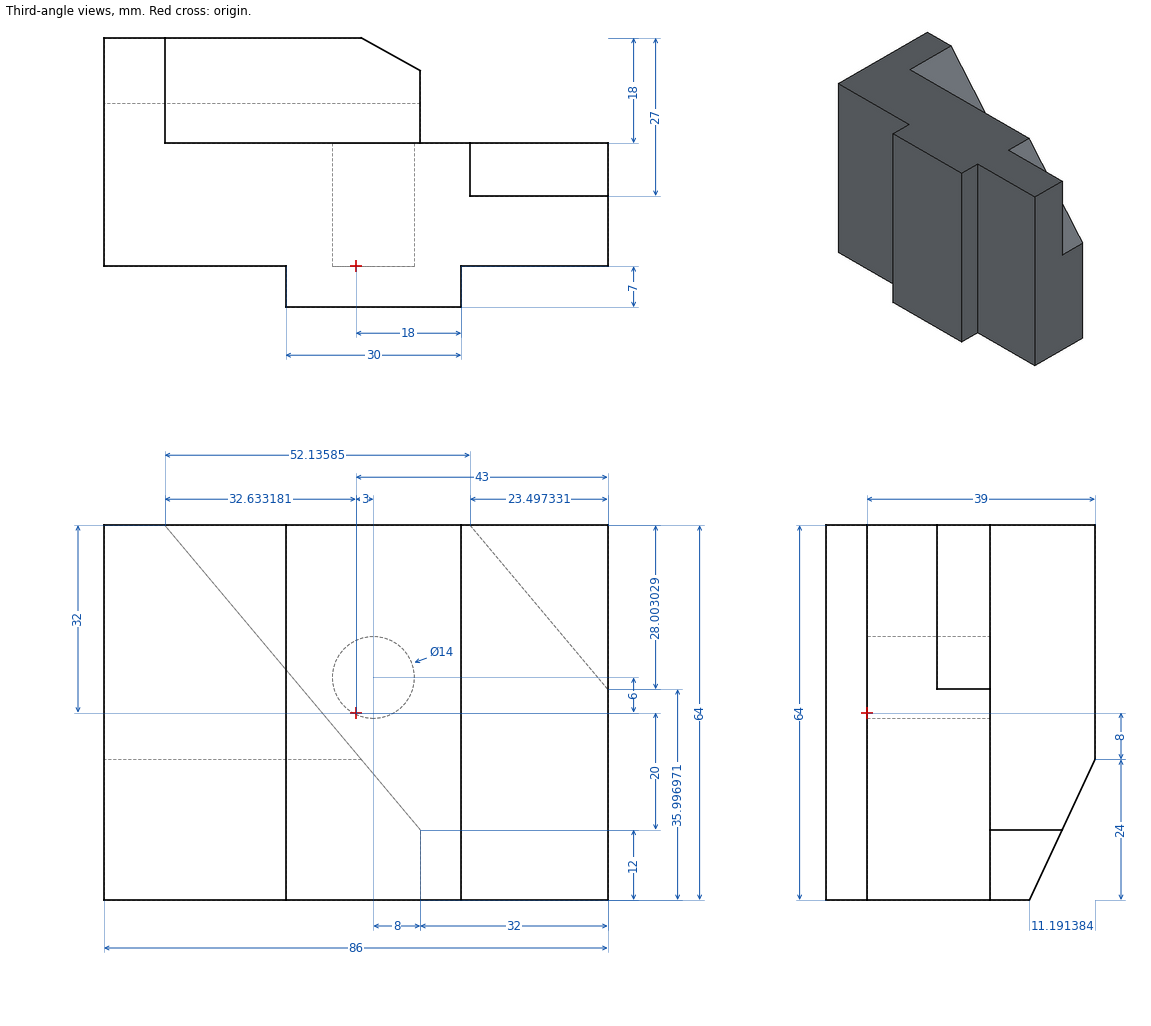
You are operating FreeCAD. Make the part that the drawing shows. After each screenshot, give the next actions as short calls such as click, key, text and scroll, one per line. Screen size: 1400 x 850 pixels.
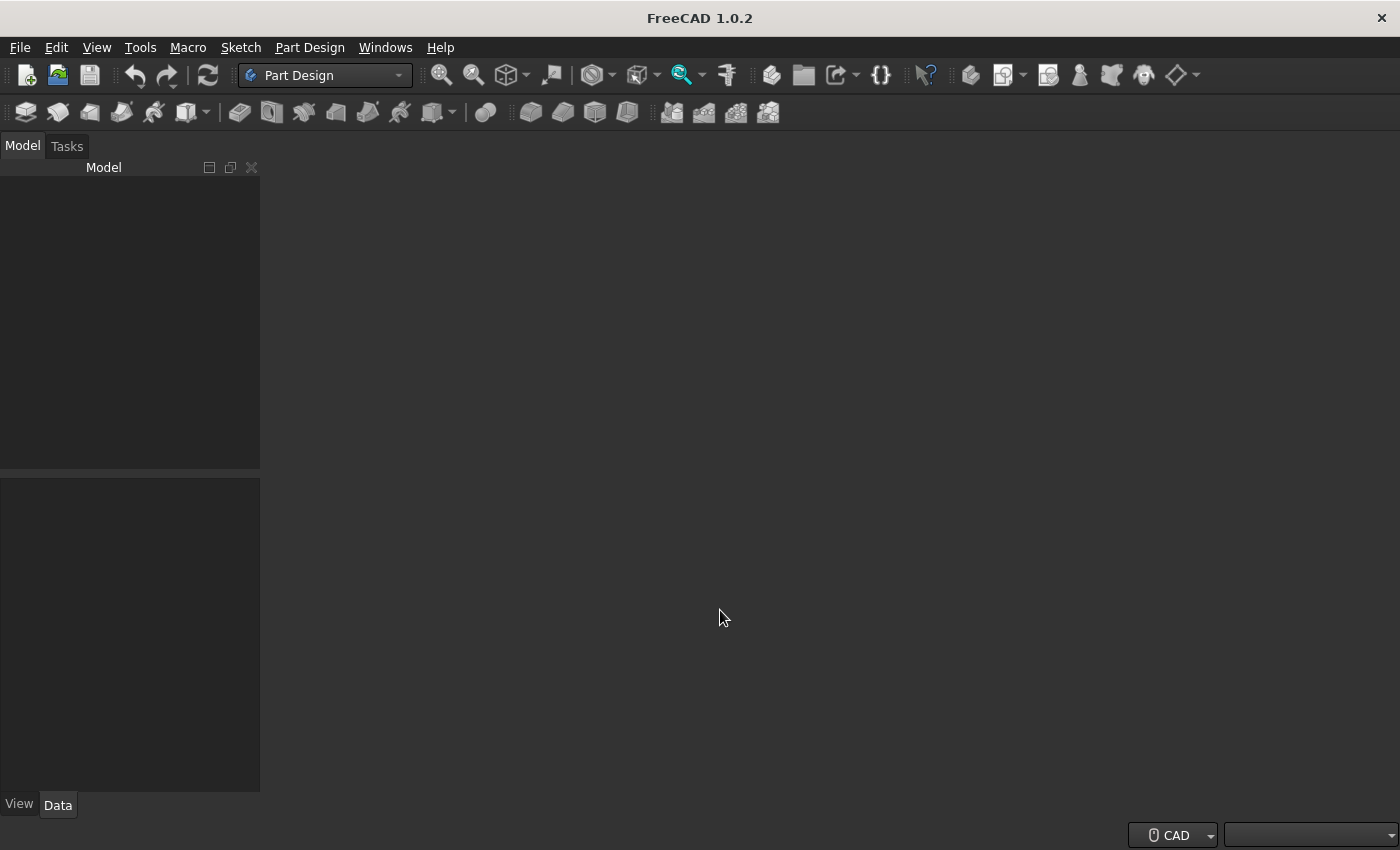
key(ctrl+n)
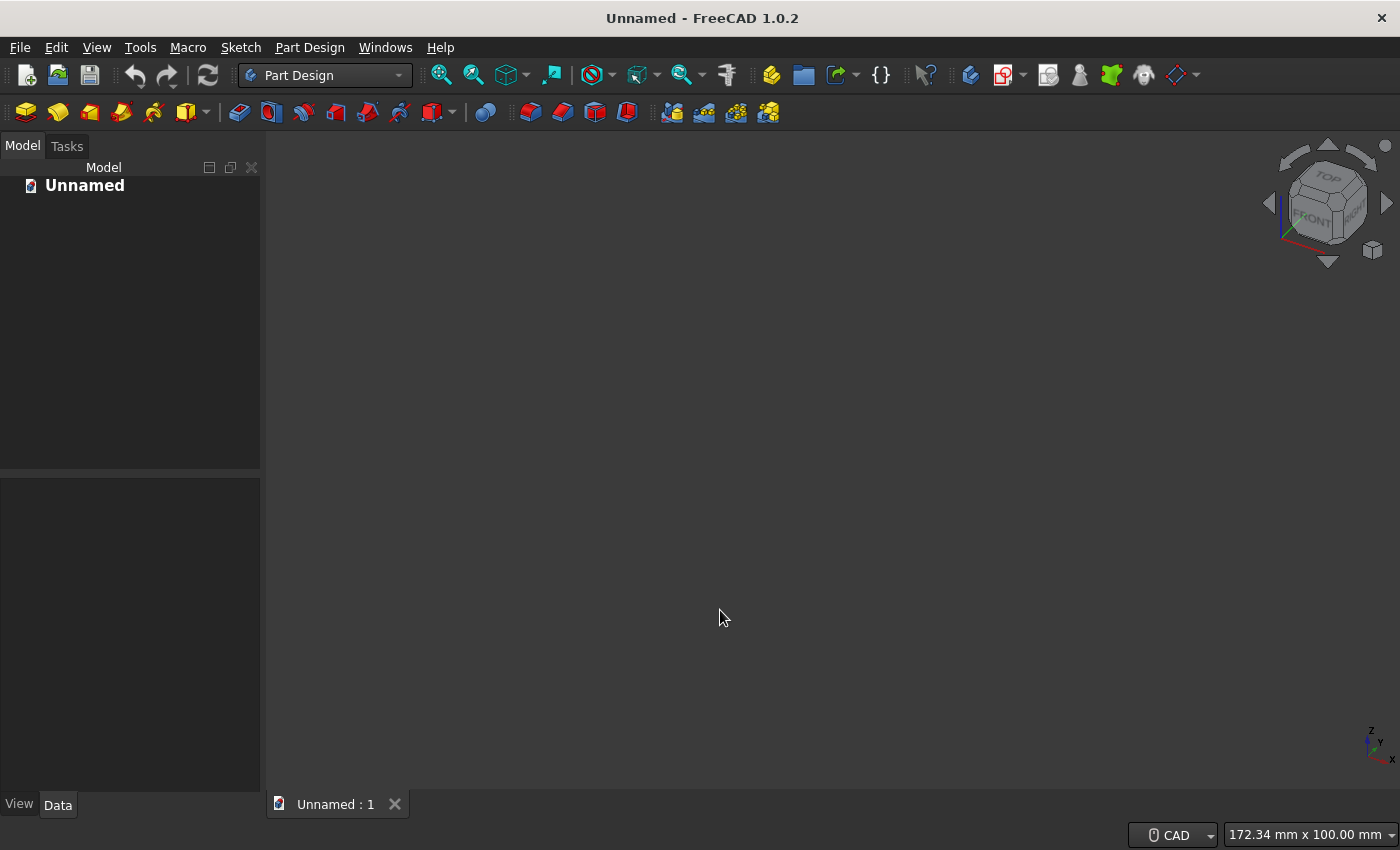
click(1004, 76)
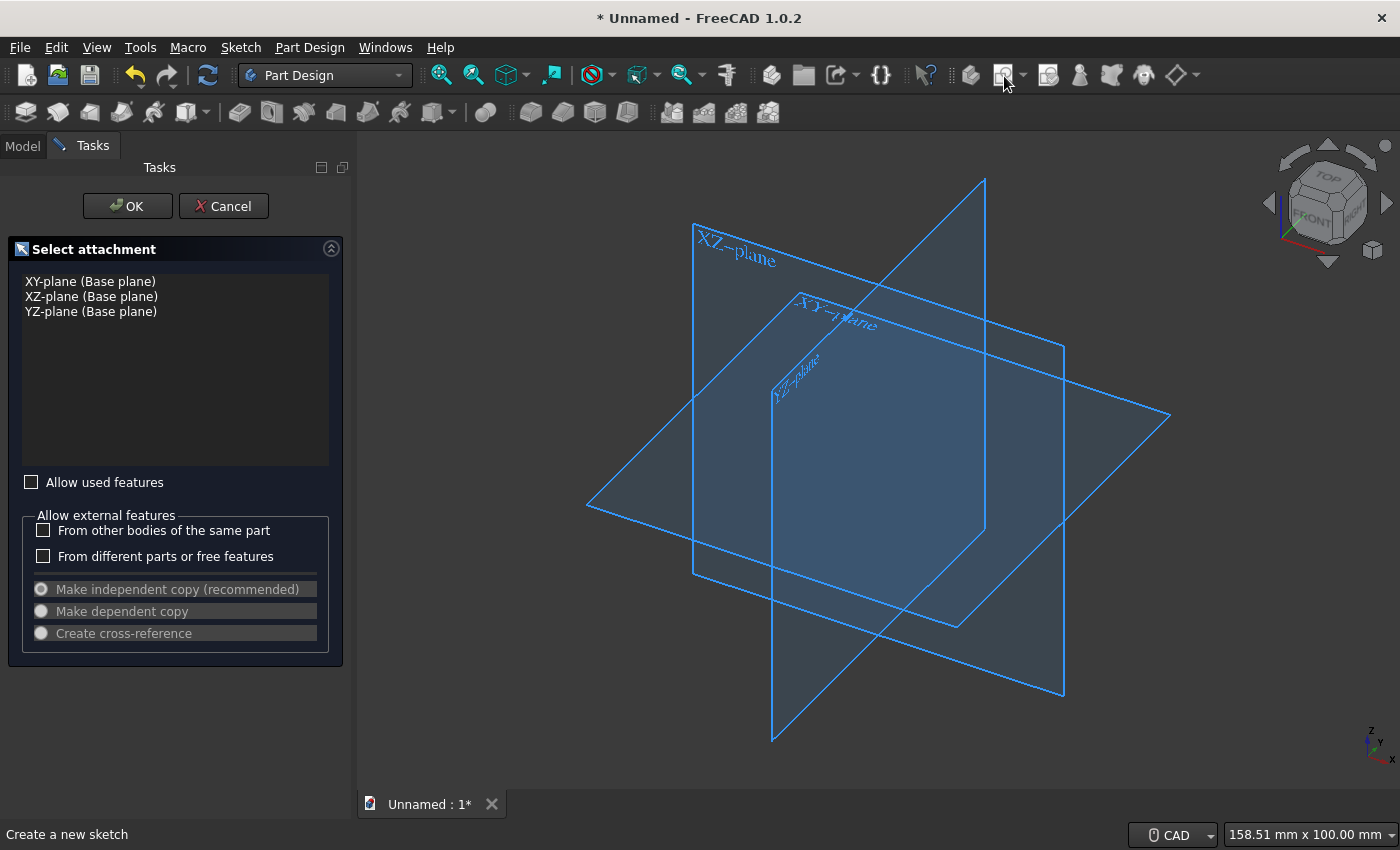
click(82, 296)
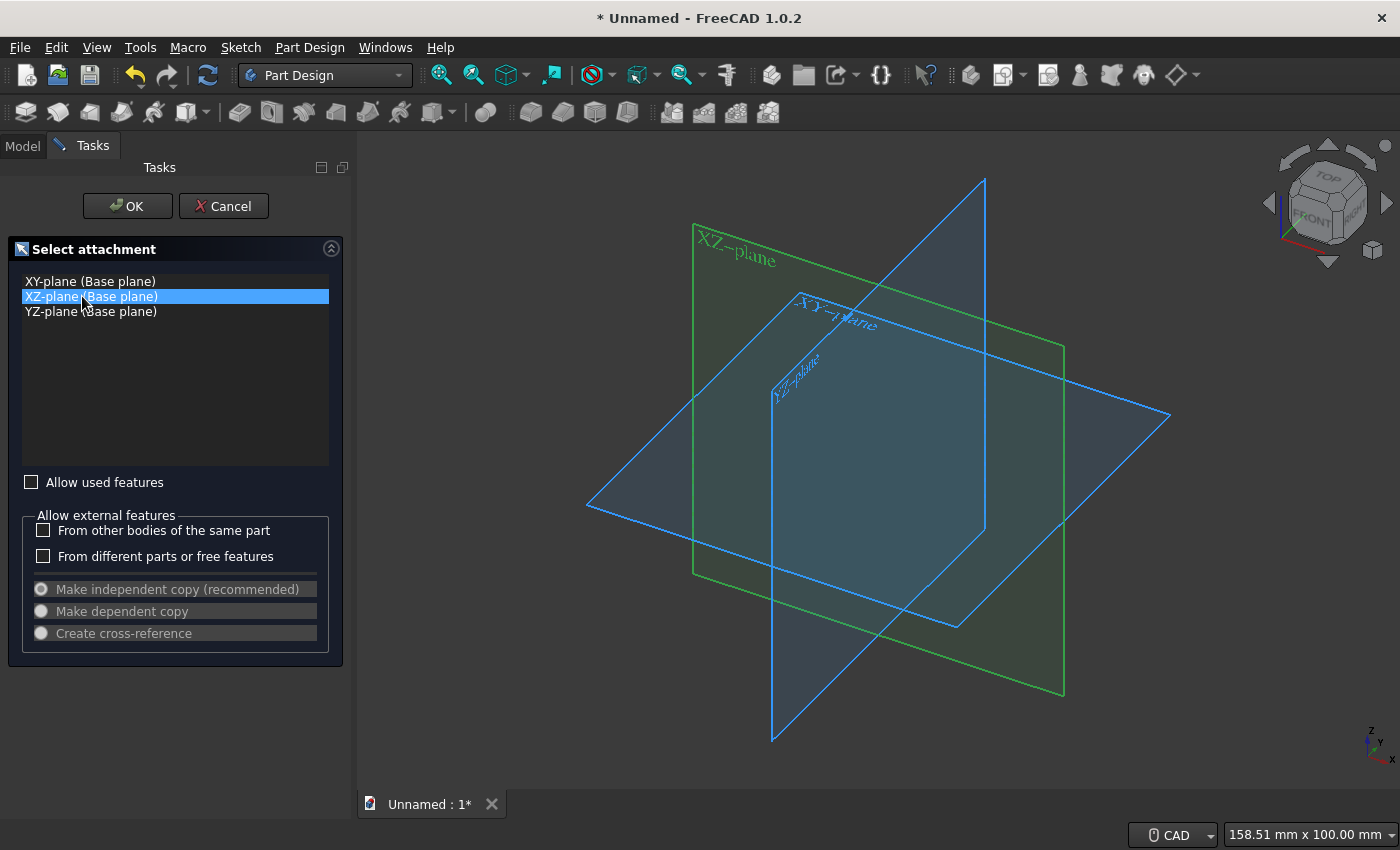
click(128, 206)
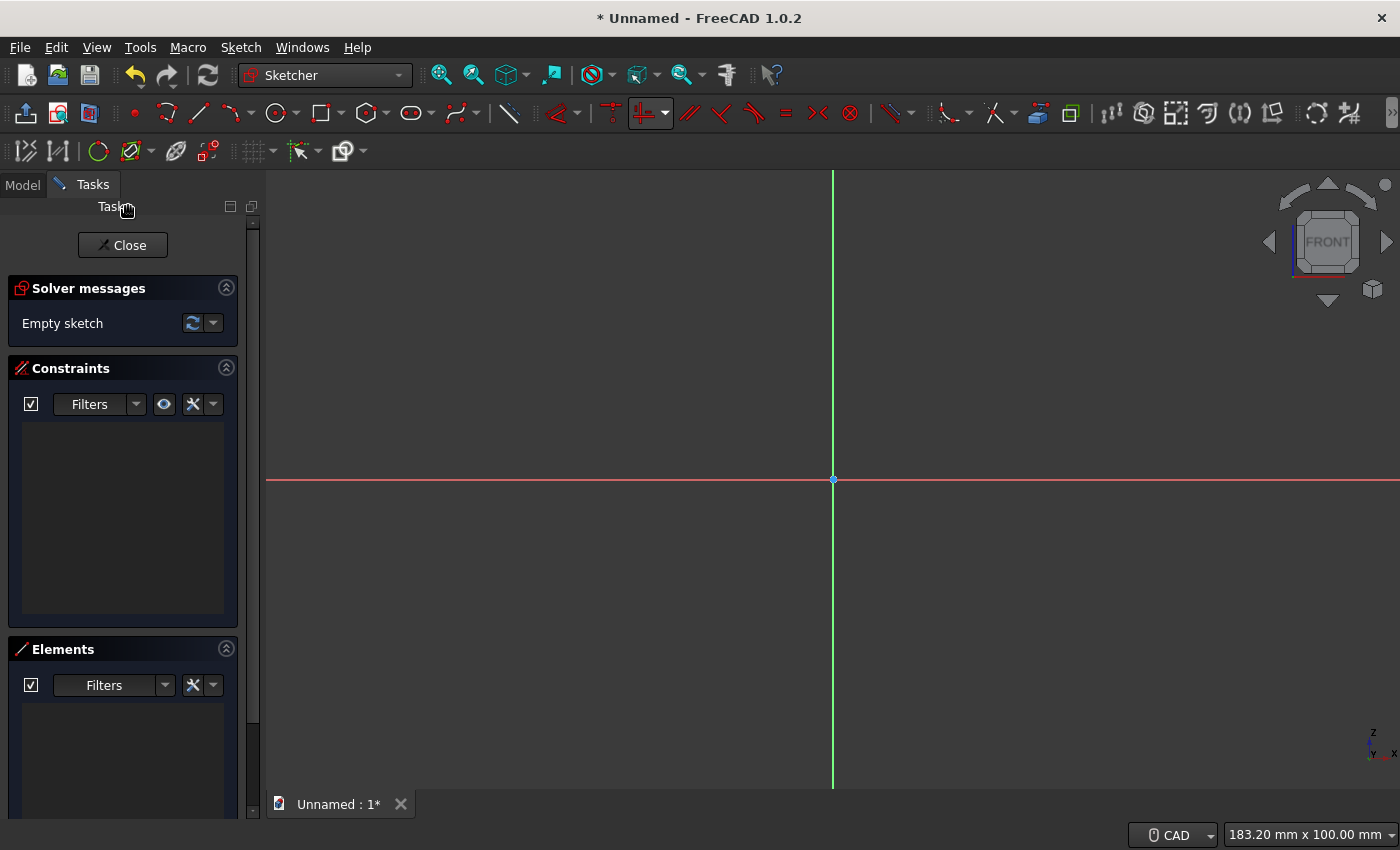
key(g)
key(v)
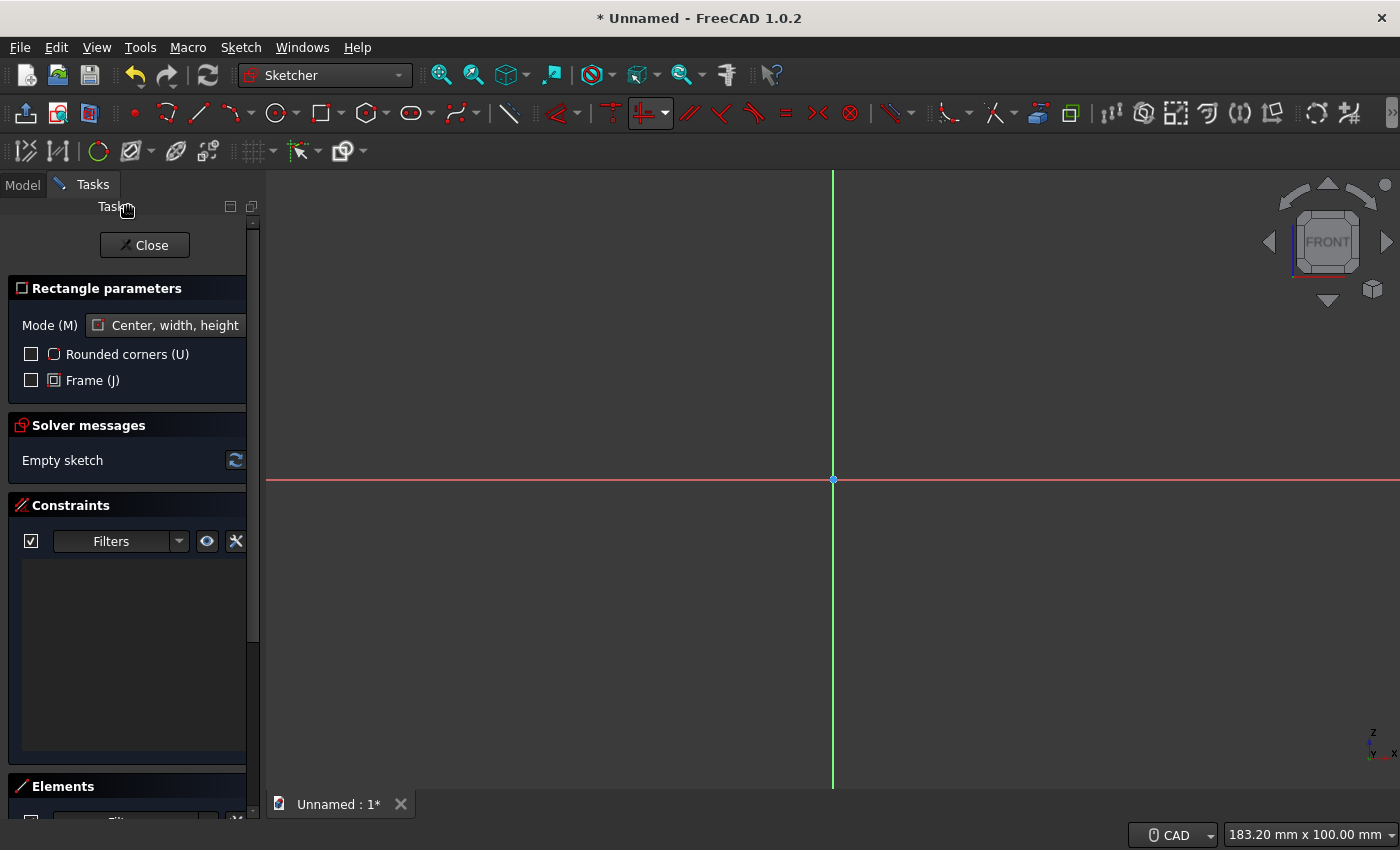
click(833, 480)
move(1099, 281)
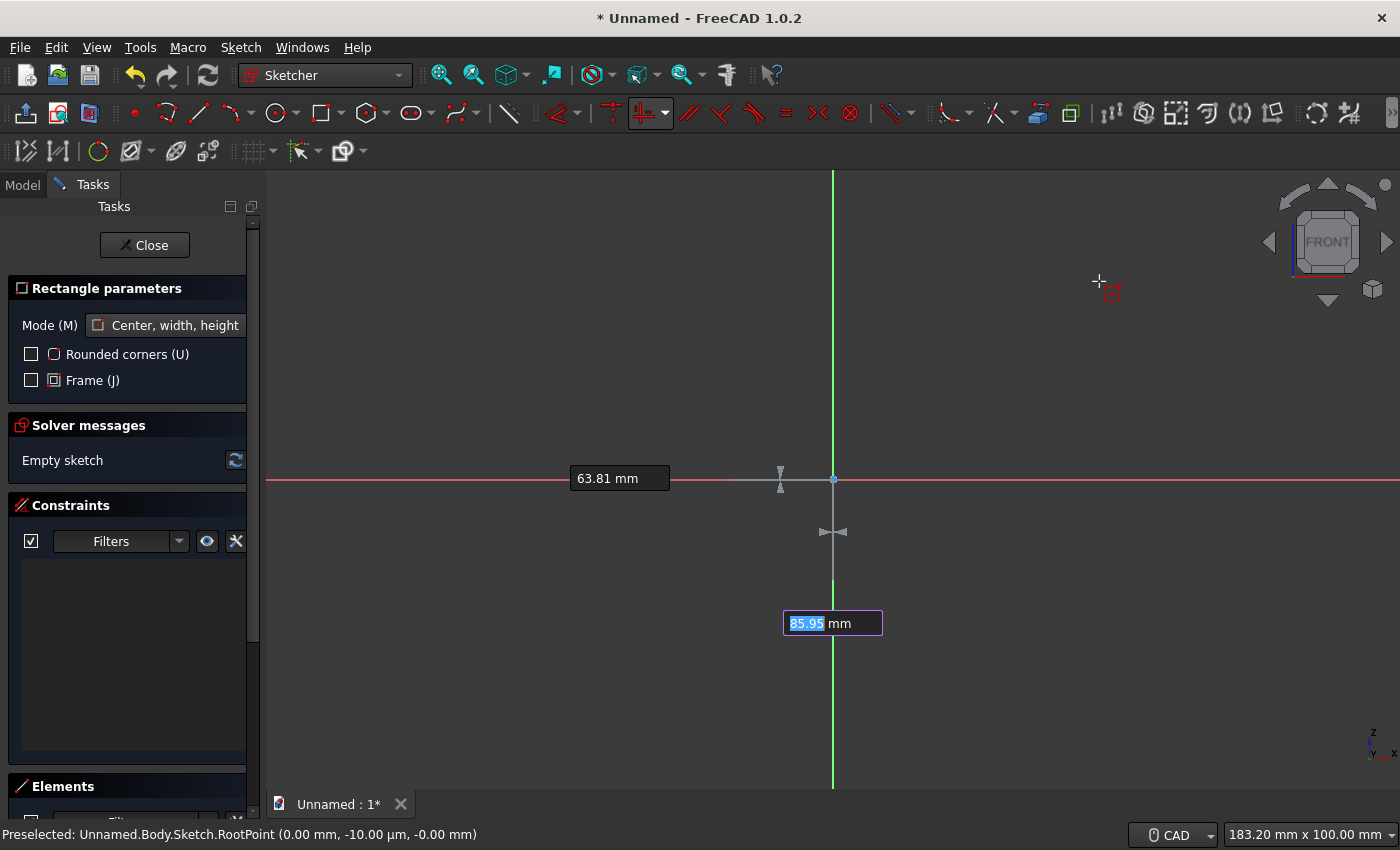
text(86)
key(Tab)
text(64)
key(Return)
key(Escape)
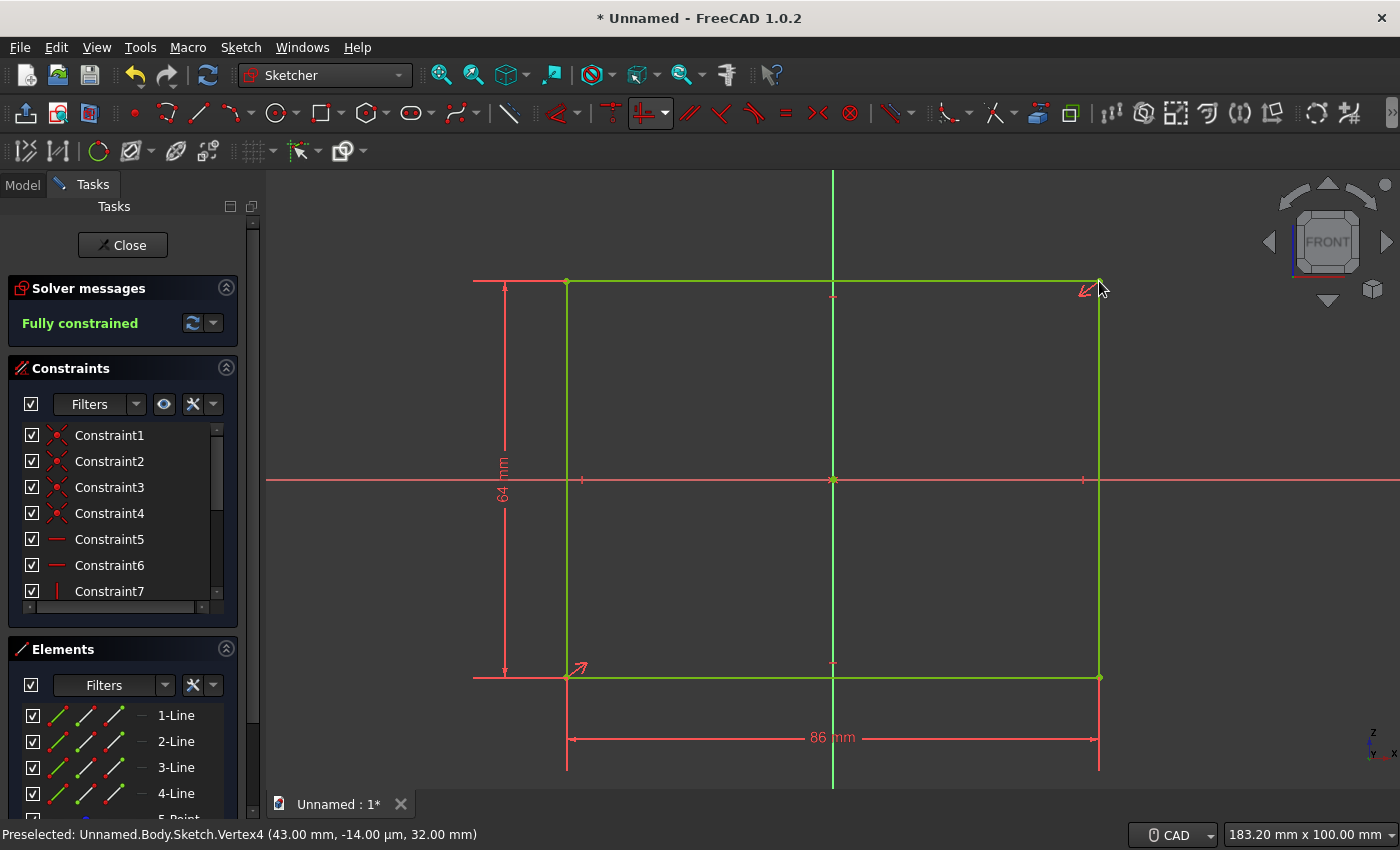
click(123, 245)